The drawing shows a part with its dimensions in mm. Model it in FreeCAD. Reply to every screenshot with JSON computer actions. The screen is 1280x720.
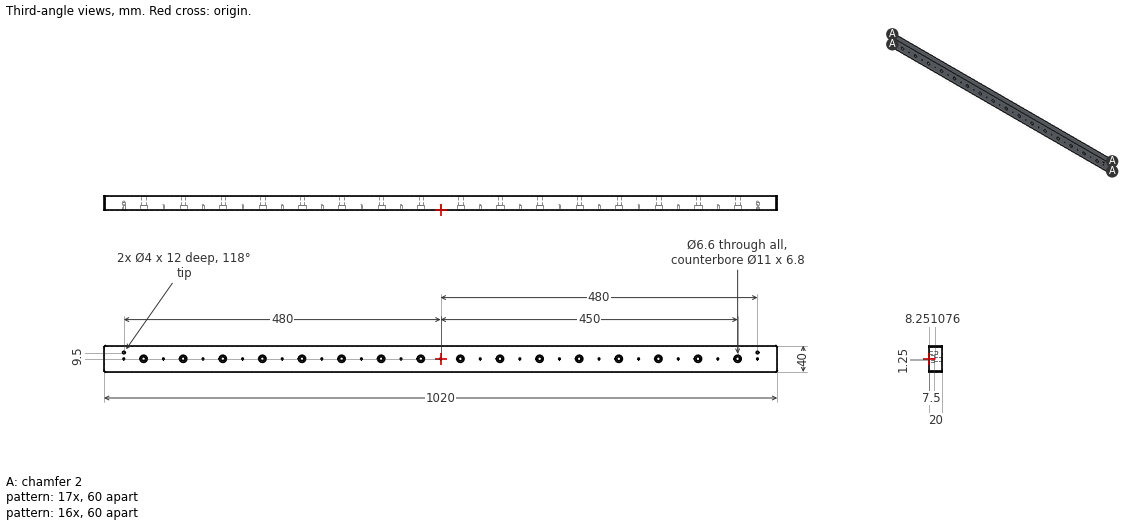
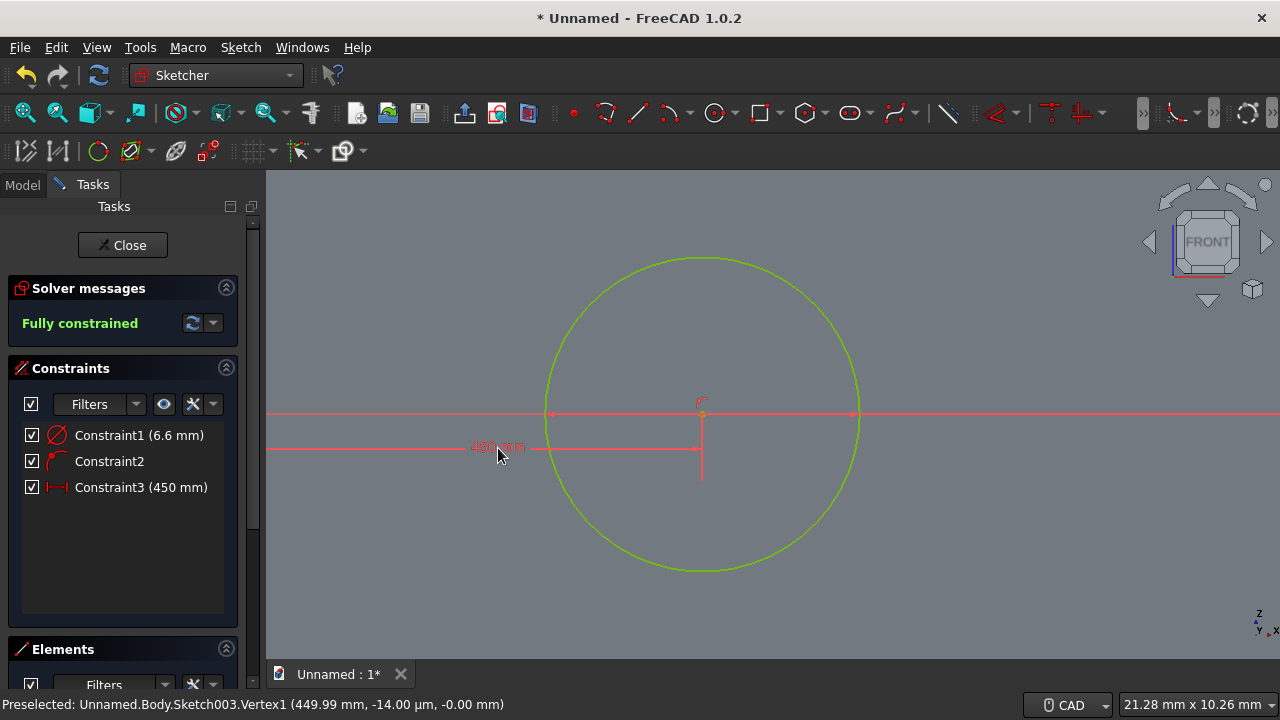
{"action": "left_click", "coordinate": [123, 245]}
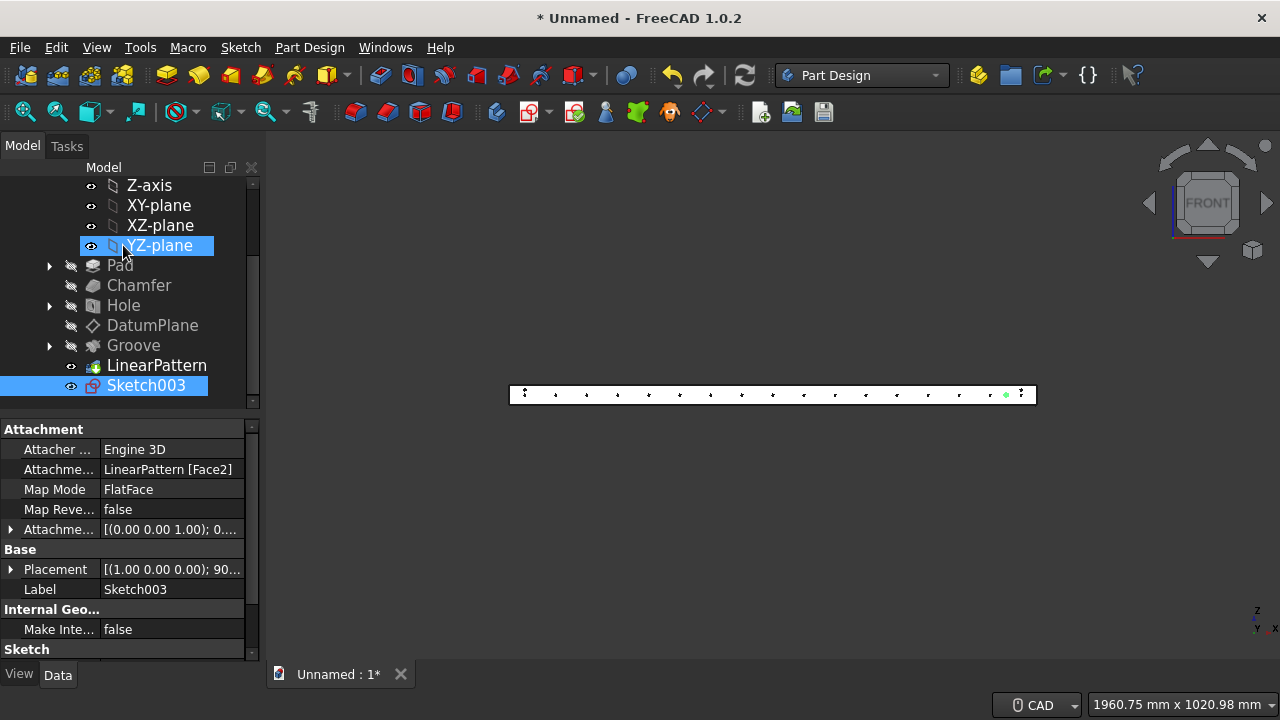
{"action": "left_click", "coordinate": [414, 76]}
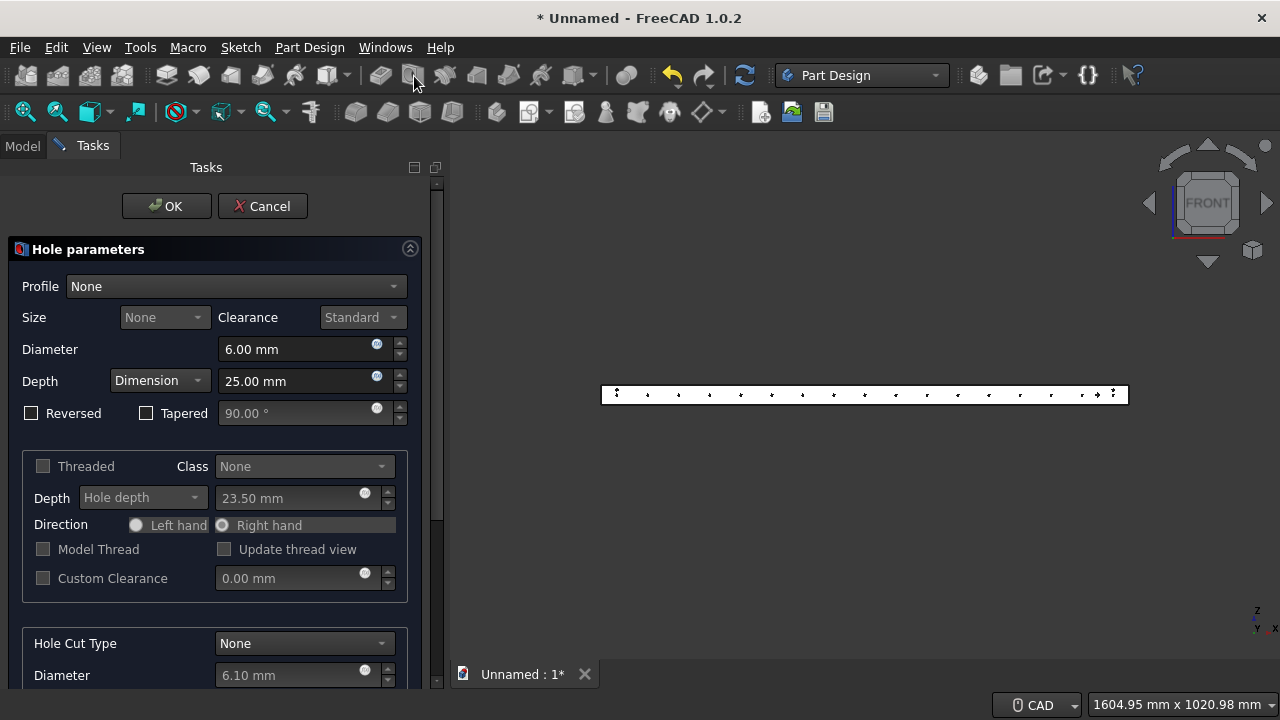
{"action": "triple_click", "coordinate": [305, 349]}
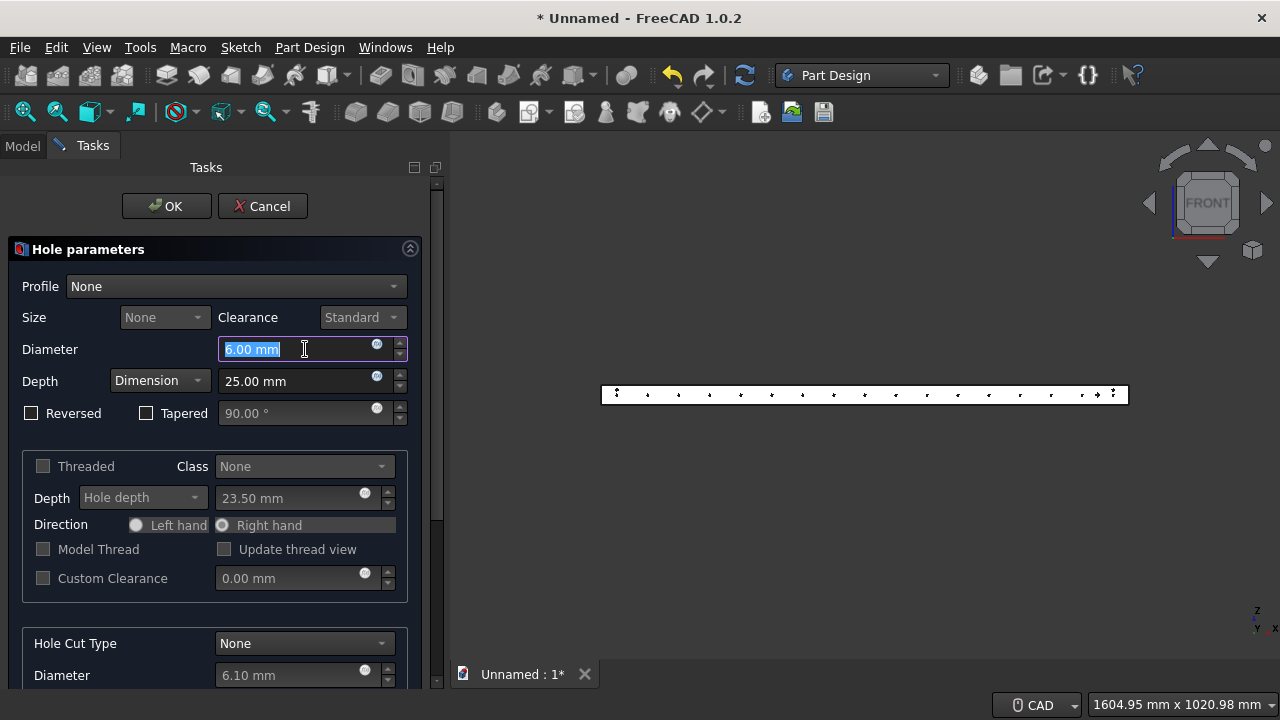
{"action": "type", "text": "6.6"}
{"action": "key", "text": "Tab"}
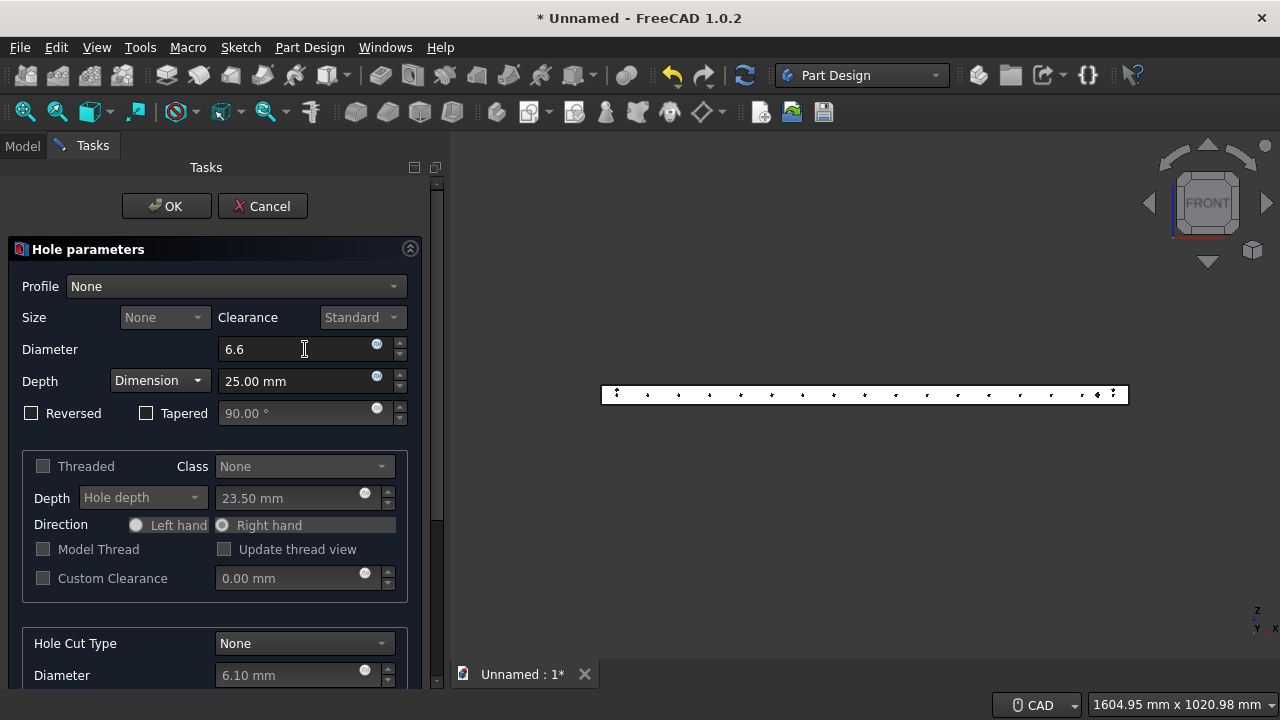
{"action": "left_click", "coordinate": [161, 380]}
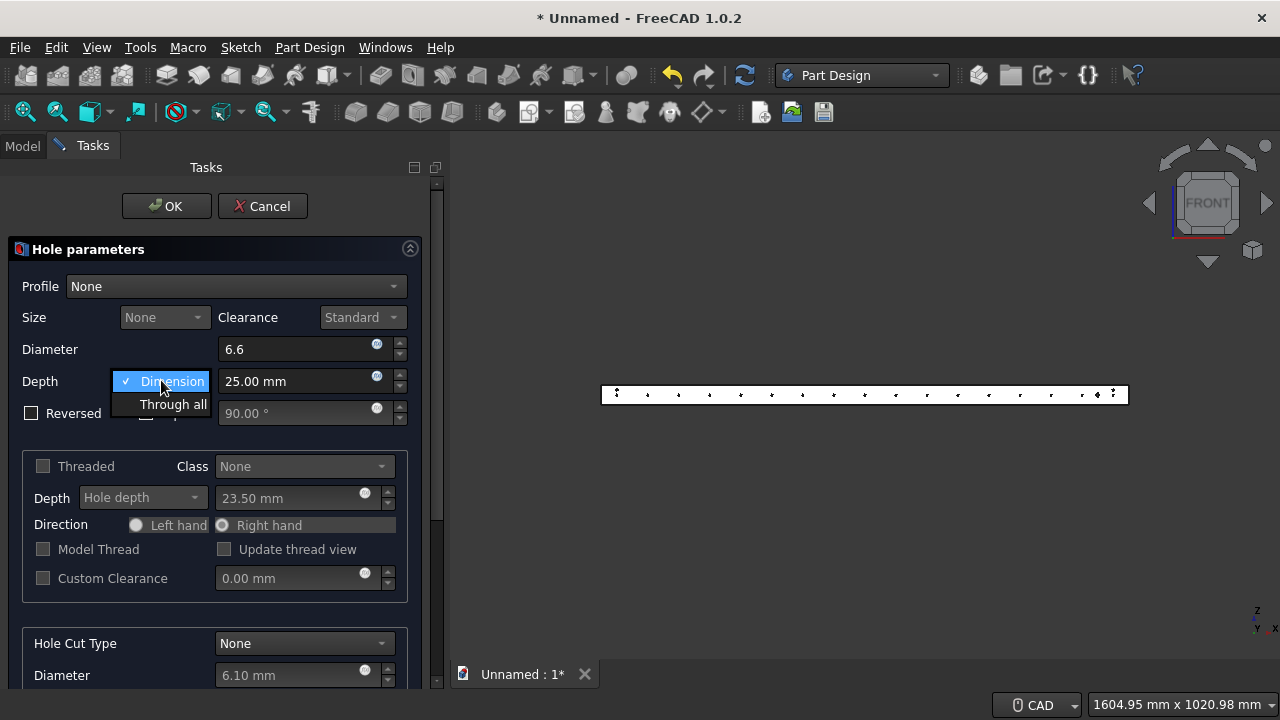
{"action": "left_click", "coordinate": [160, 404]}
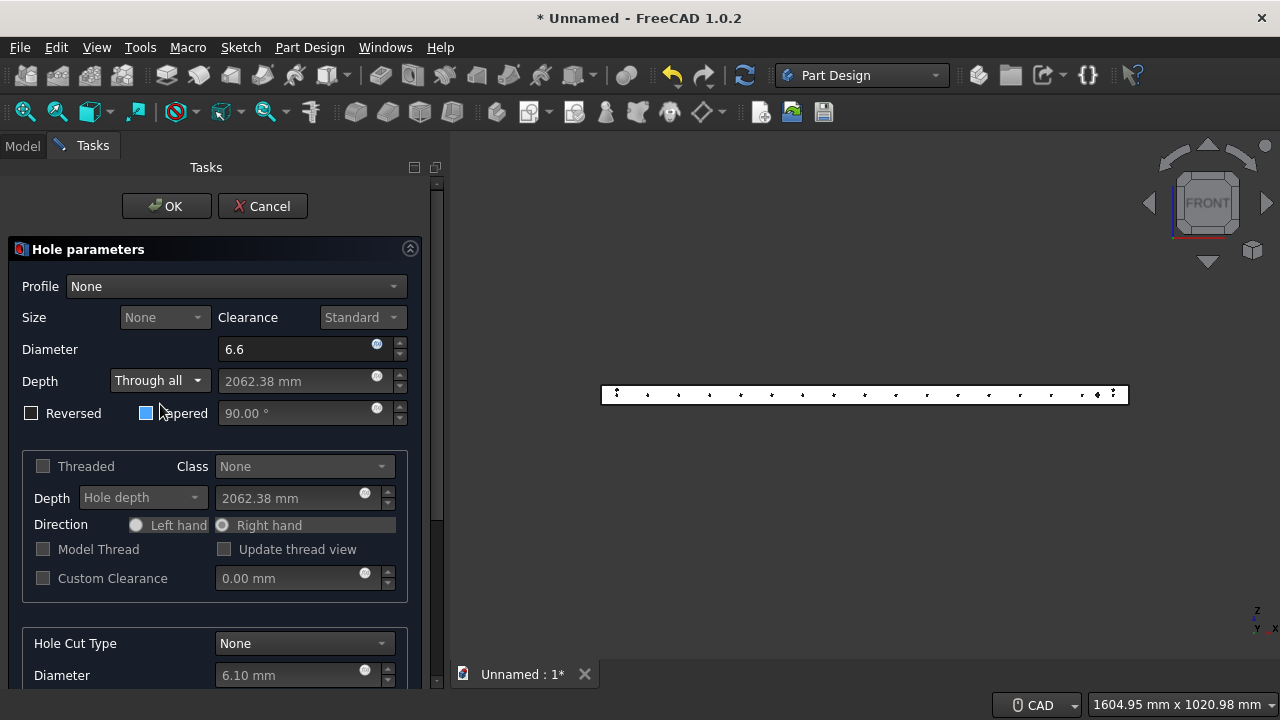
{"action": "left_click", "coordinate": [306, 644]}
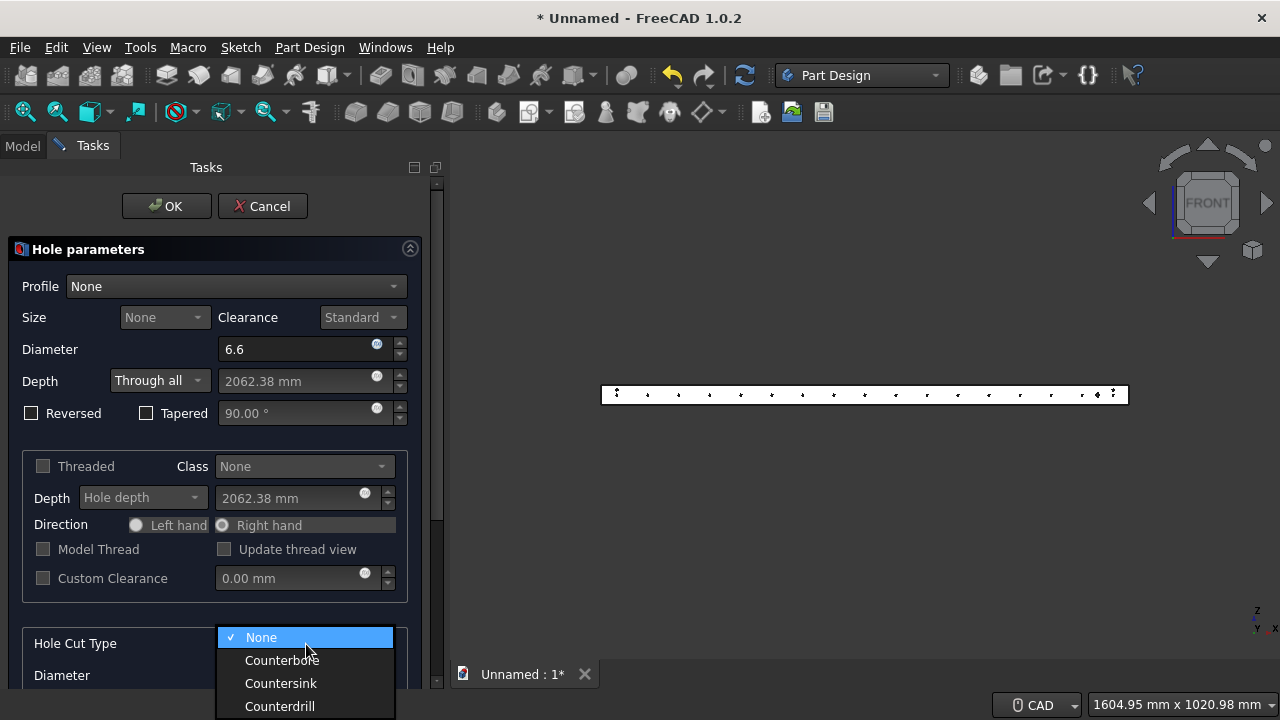
{"action": "left_click", "coordinate": [304, 660]}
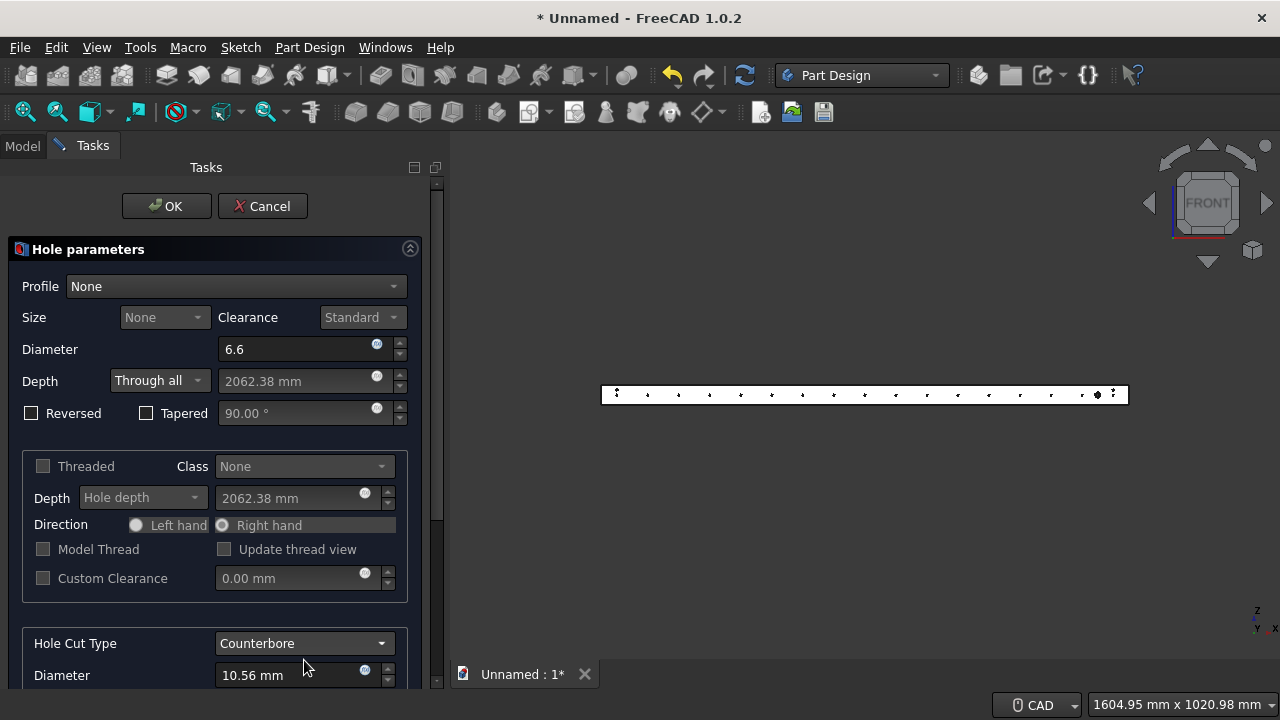
{"action": "triple_click", "coordinate": [298, 675]}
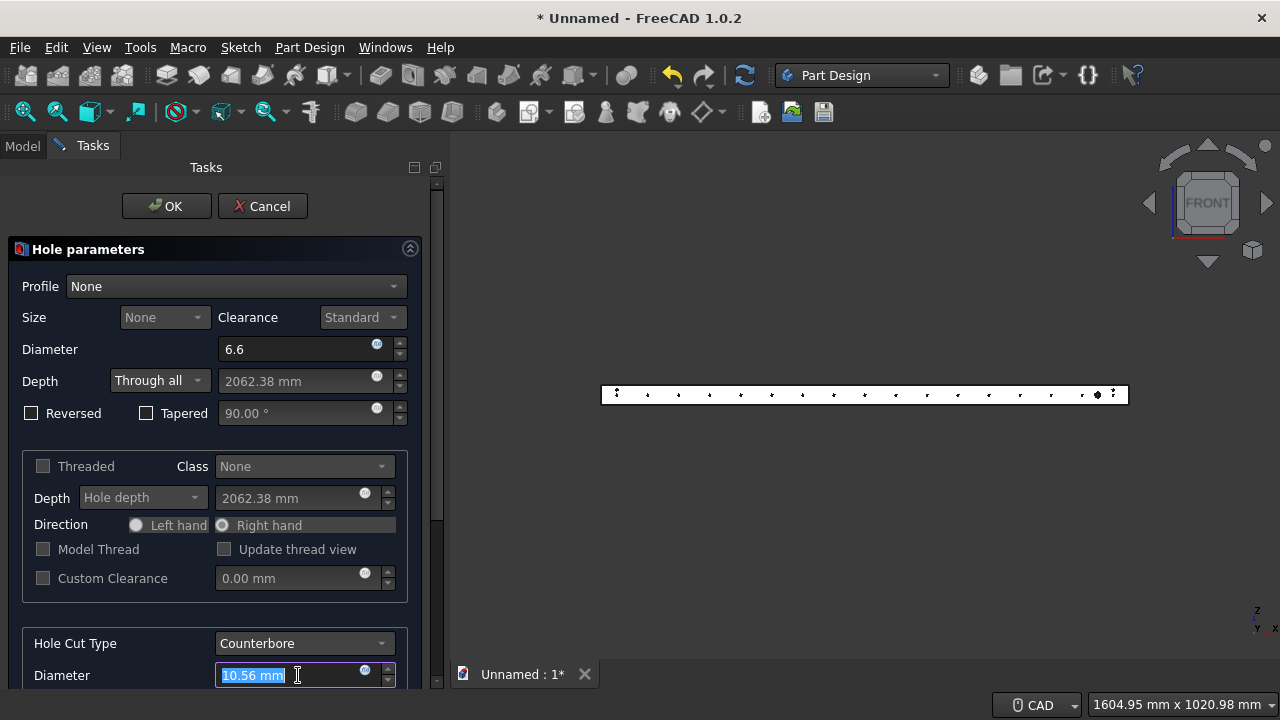
{"action": "type", "text": "11"}
{"action": "key", "text": "Tab"}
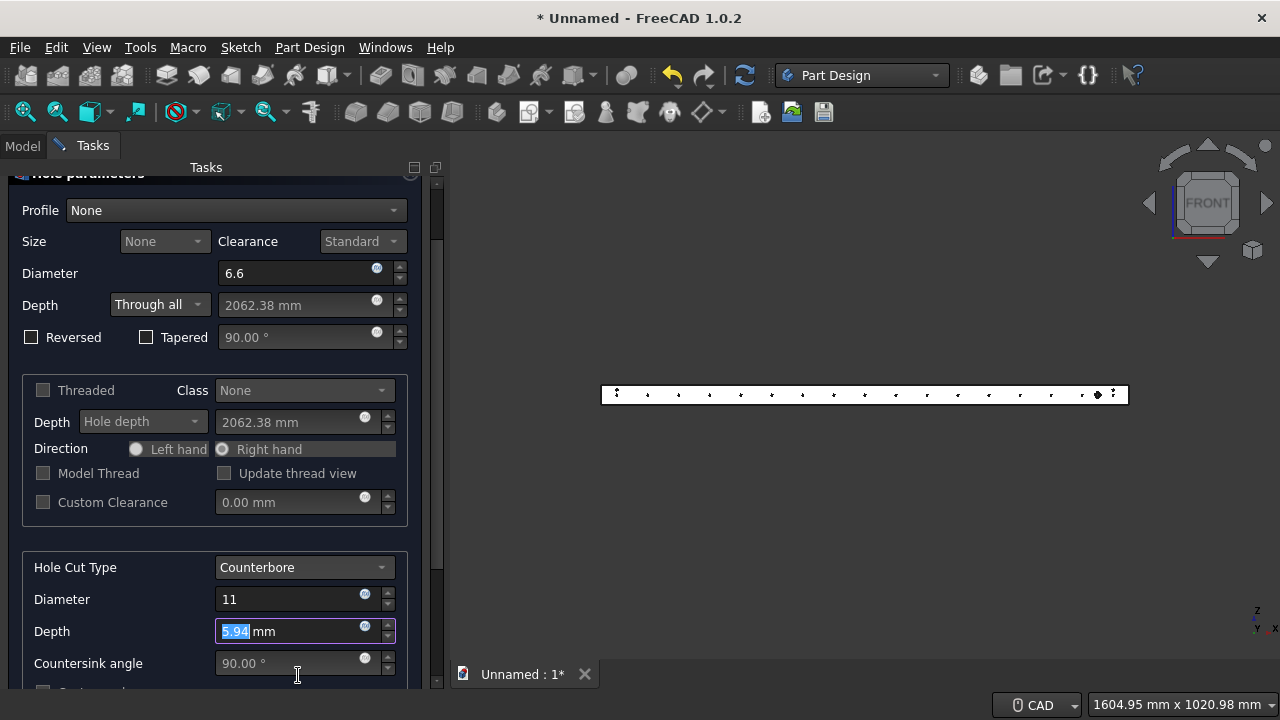
{"action": "type", "text": "6.8"}
{"action": "key", "text": "Tab"}